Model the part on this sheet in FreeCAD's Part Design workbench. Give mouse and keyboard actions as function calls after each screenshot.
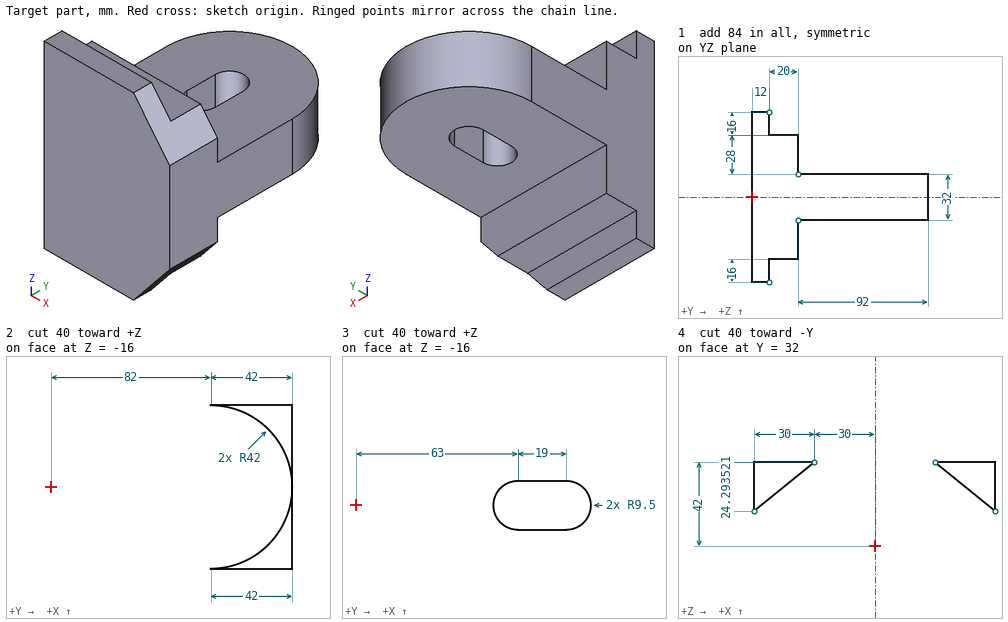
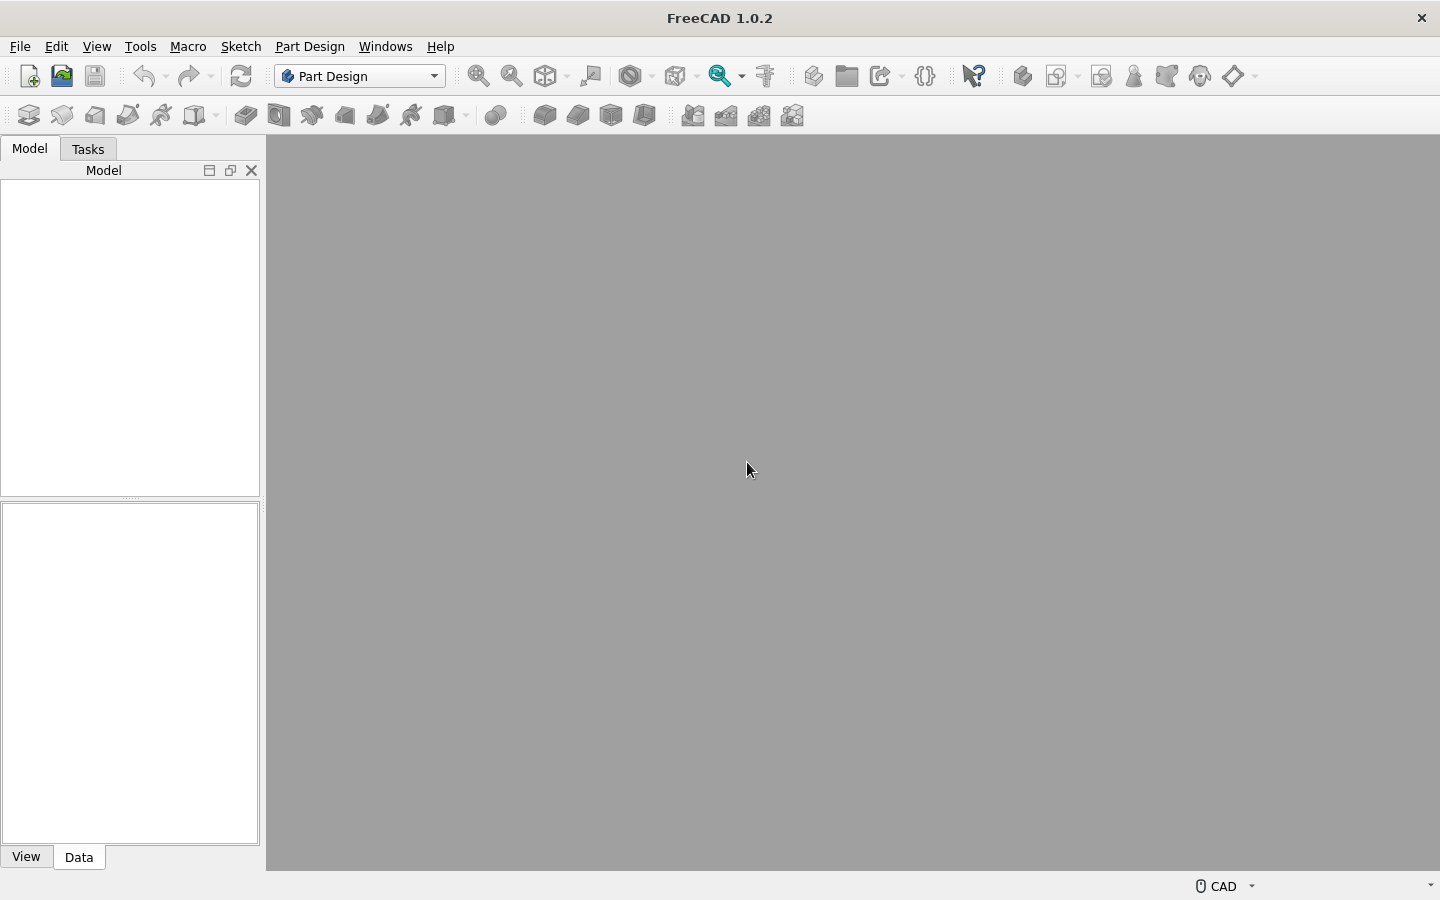
key(ctrl+n)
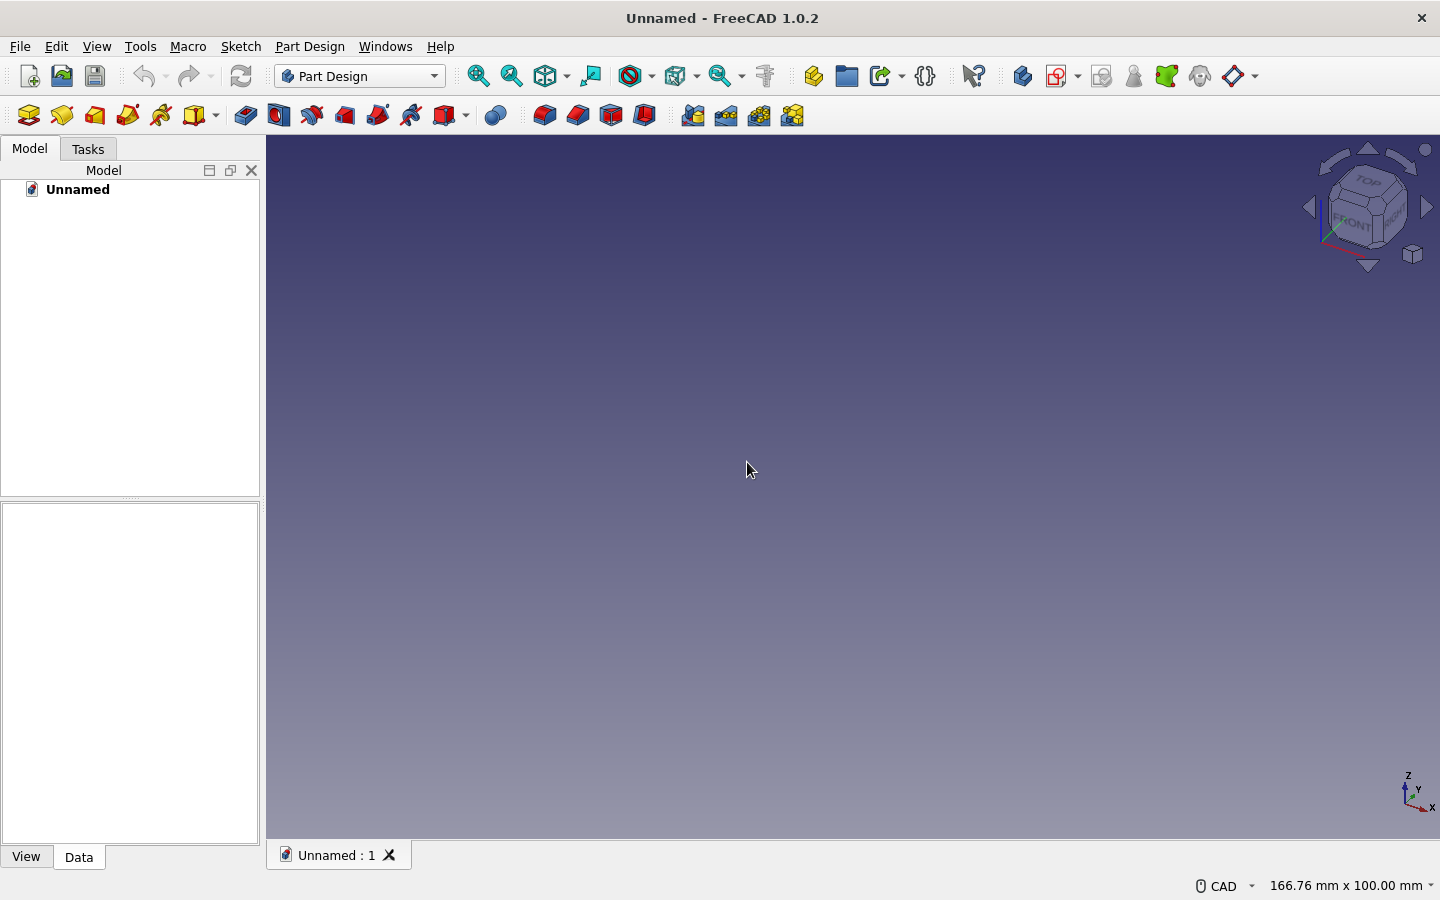
click(1056, 76)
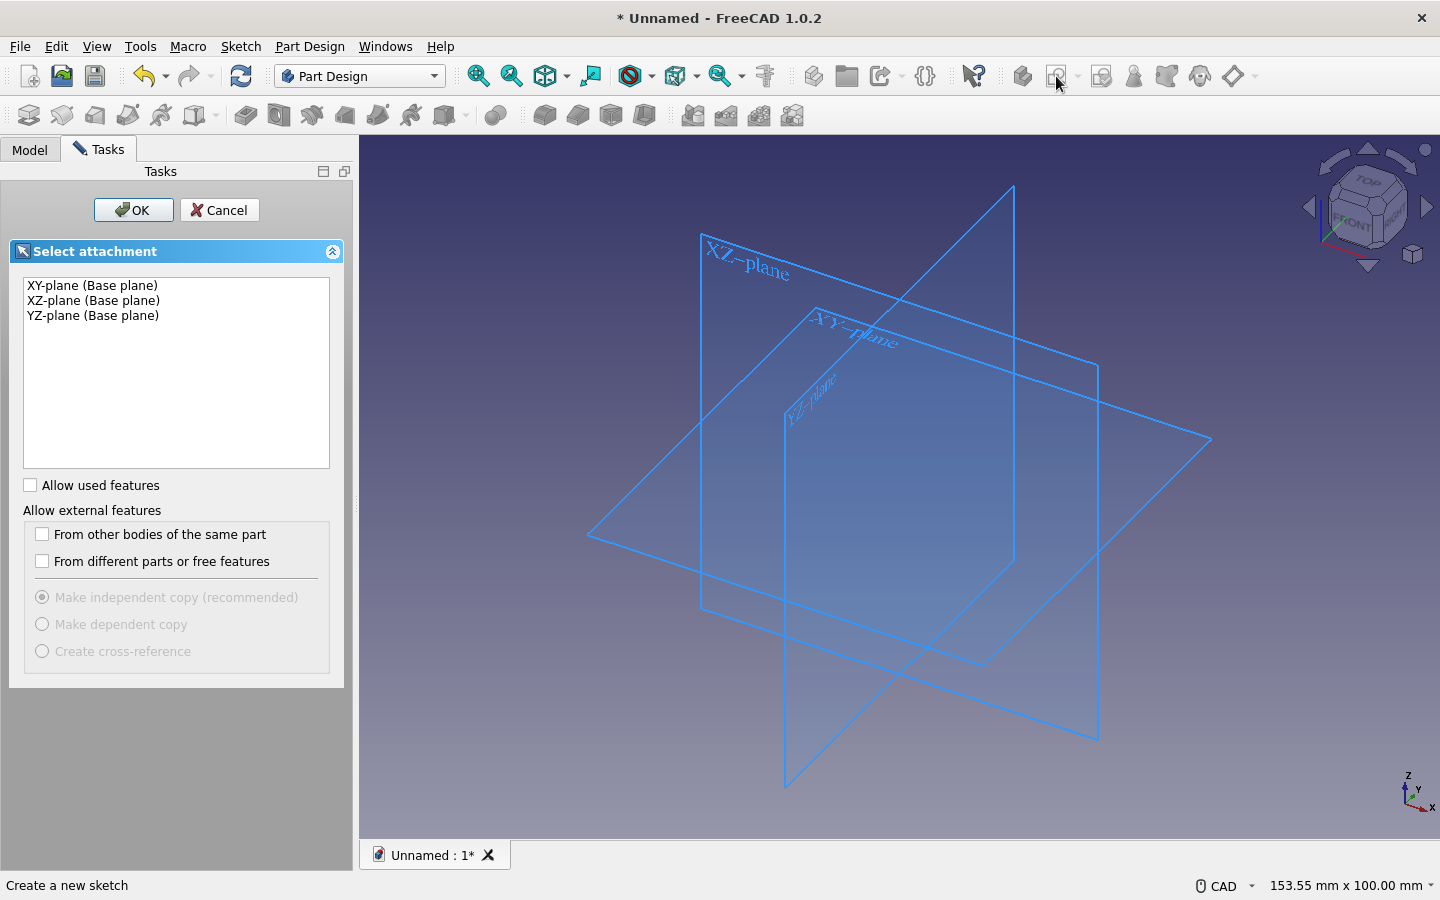
click(84, 316)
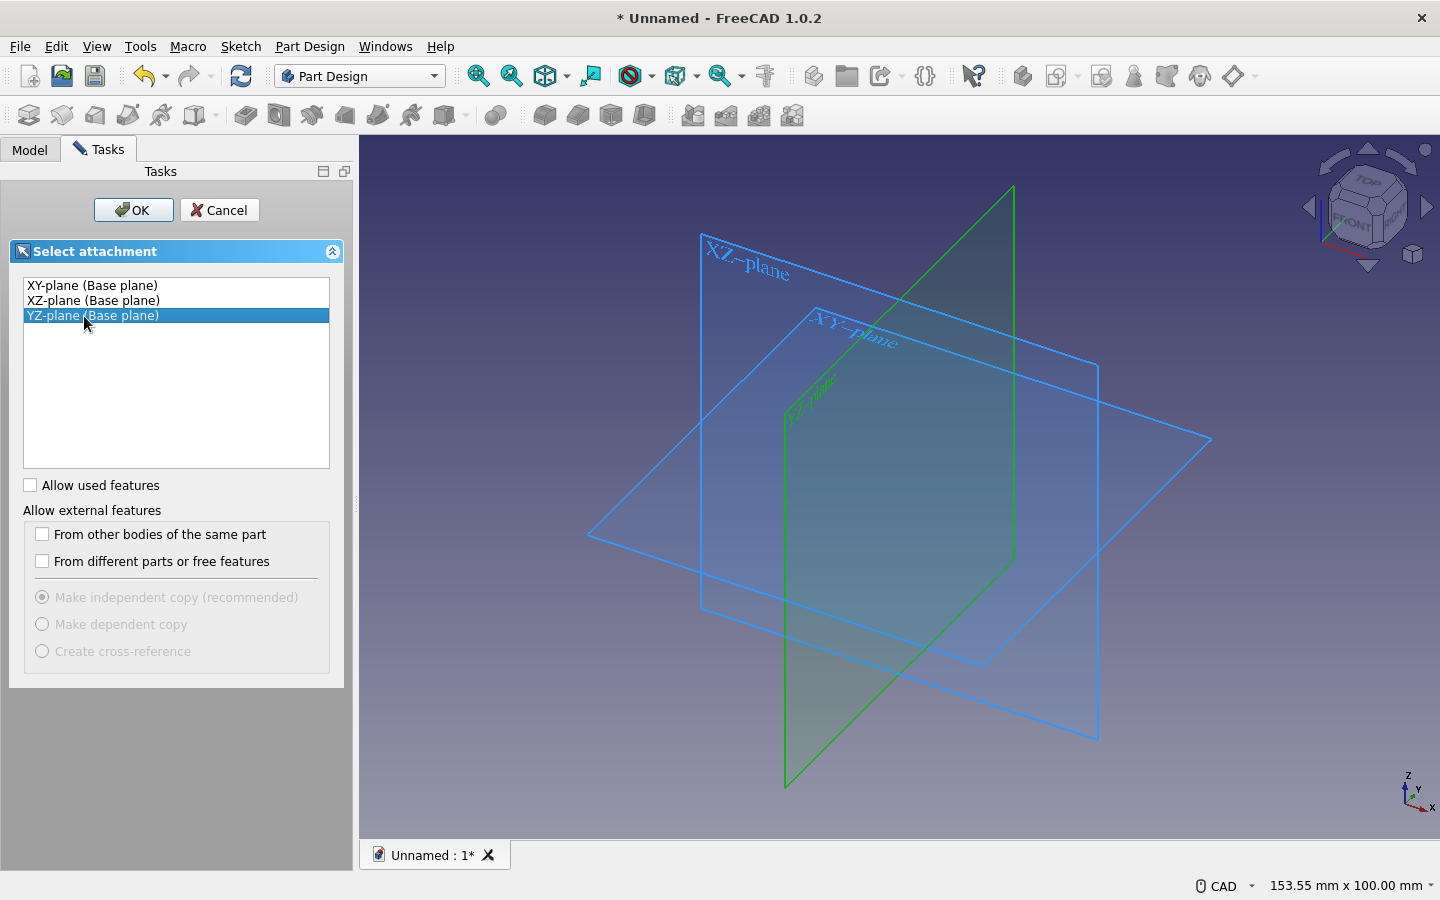
click(134, 210)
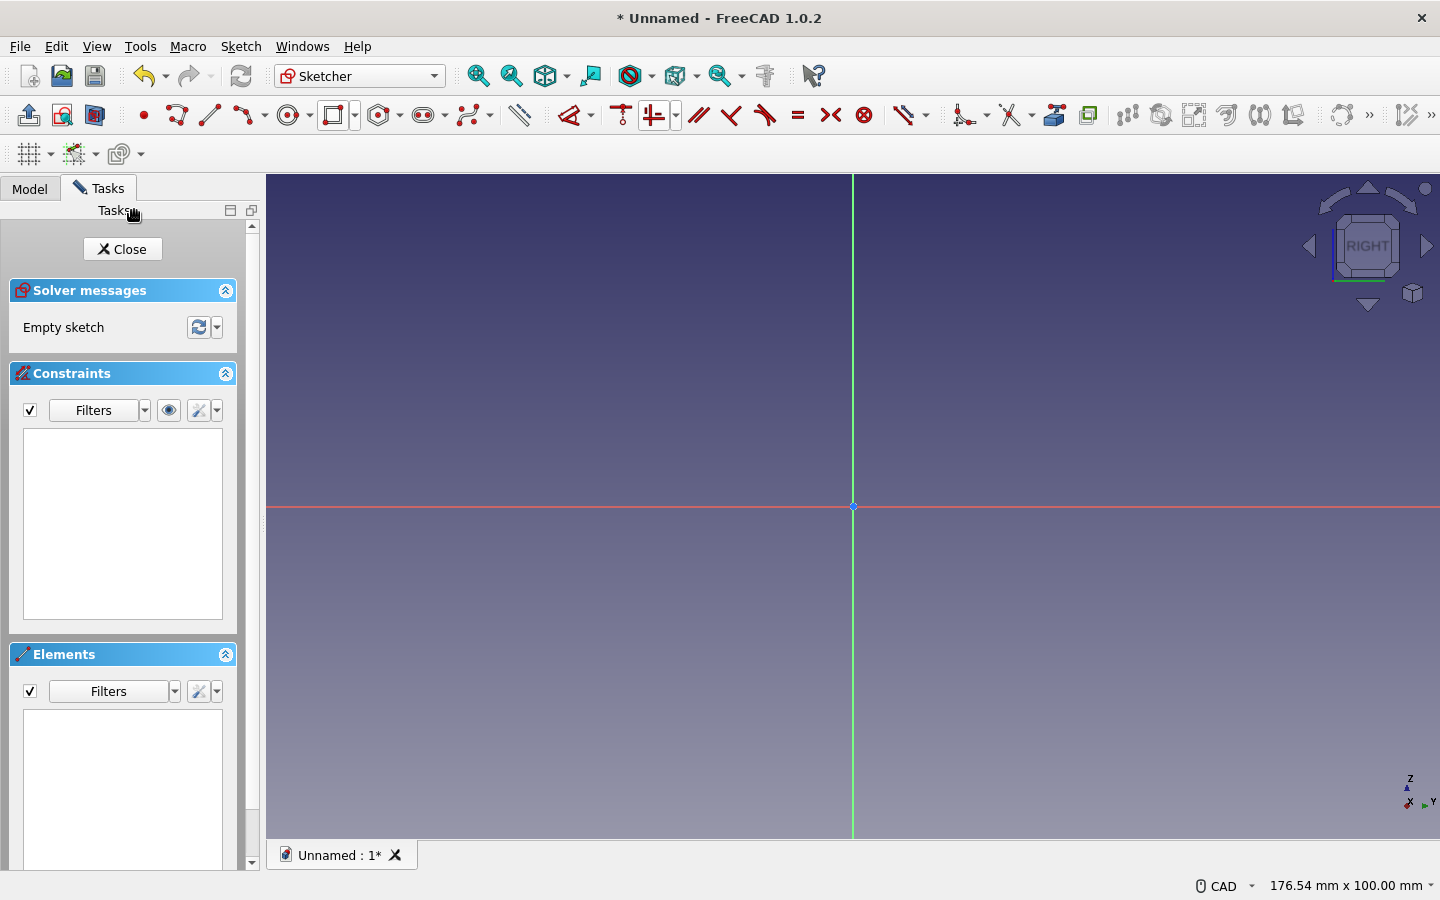
scroll(294, 506, down, 3)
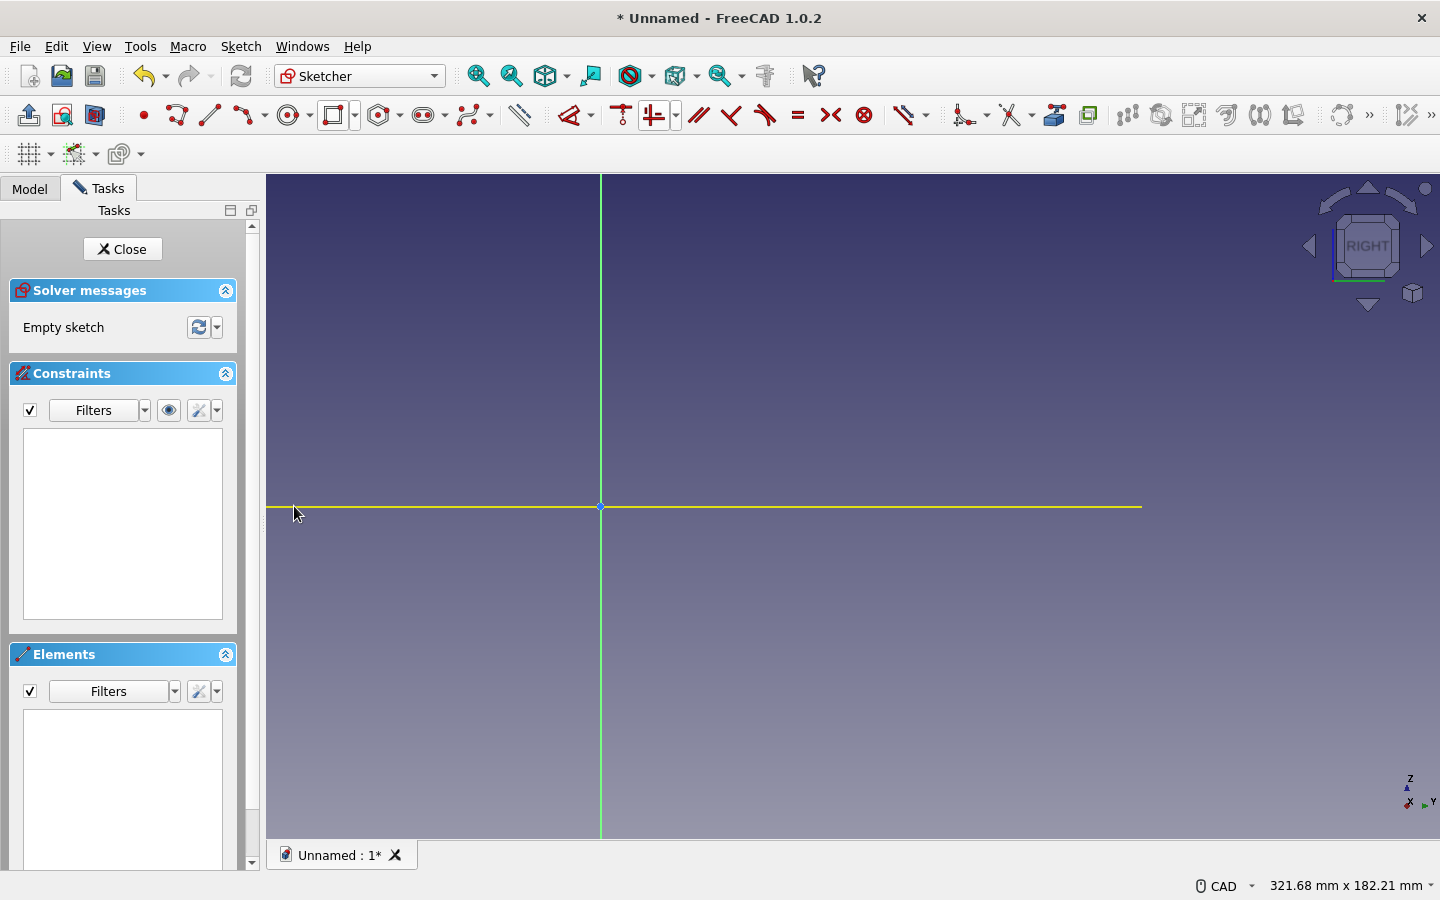
key(g)
key(m)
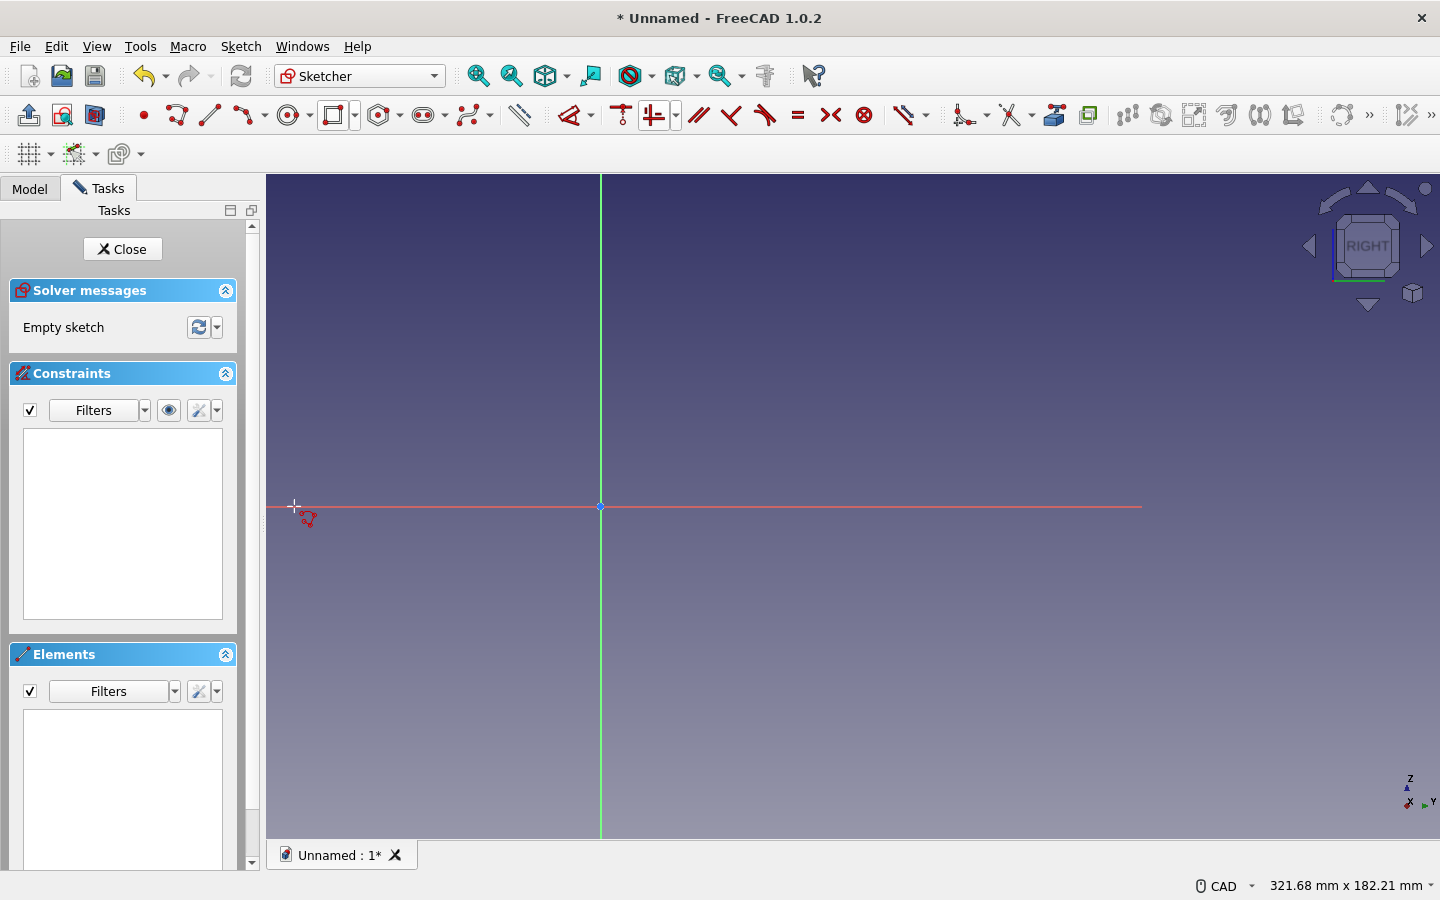
click(718, 565)
click(1053, 565)
click(1053, 448)
click(718, 448)
click(718, 346)
click(645, 346)
click(645, 288)
click(601, 288)
click(610, 725)
click(645, 725)
click(645, 667)
click(718, 667)
click(718, 566)
key(Escape)
key(Escape)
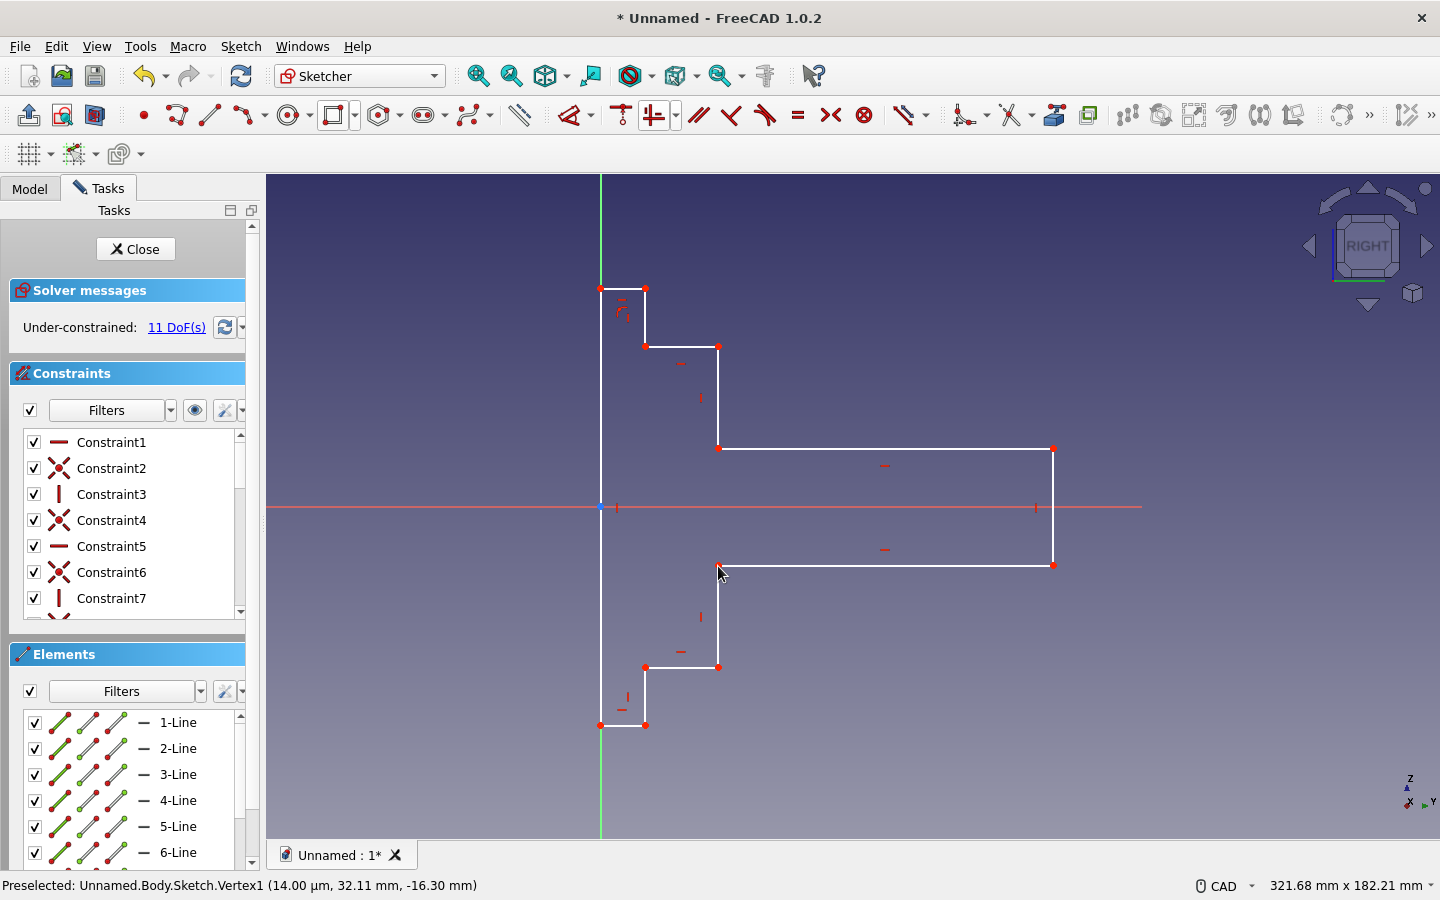
click(718, 566)